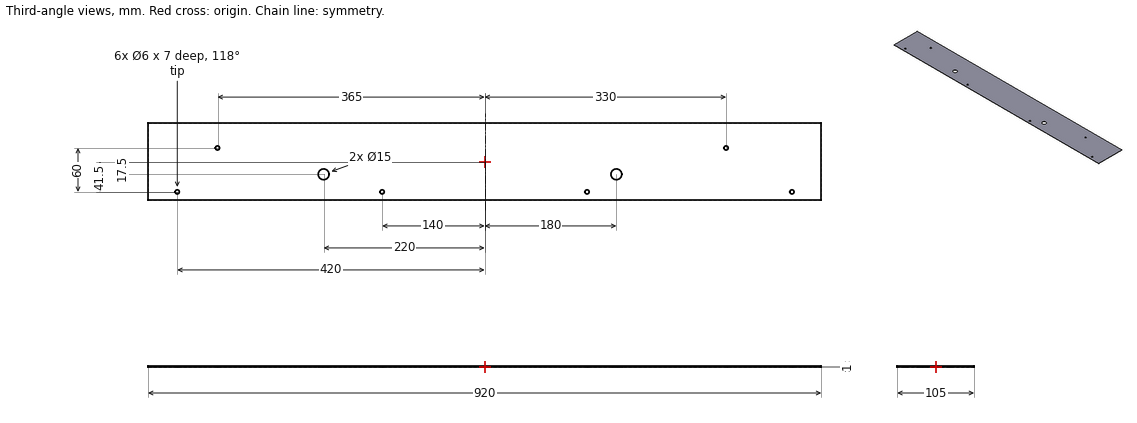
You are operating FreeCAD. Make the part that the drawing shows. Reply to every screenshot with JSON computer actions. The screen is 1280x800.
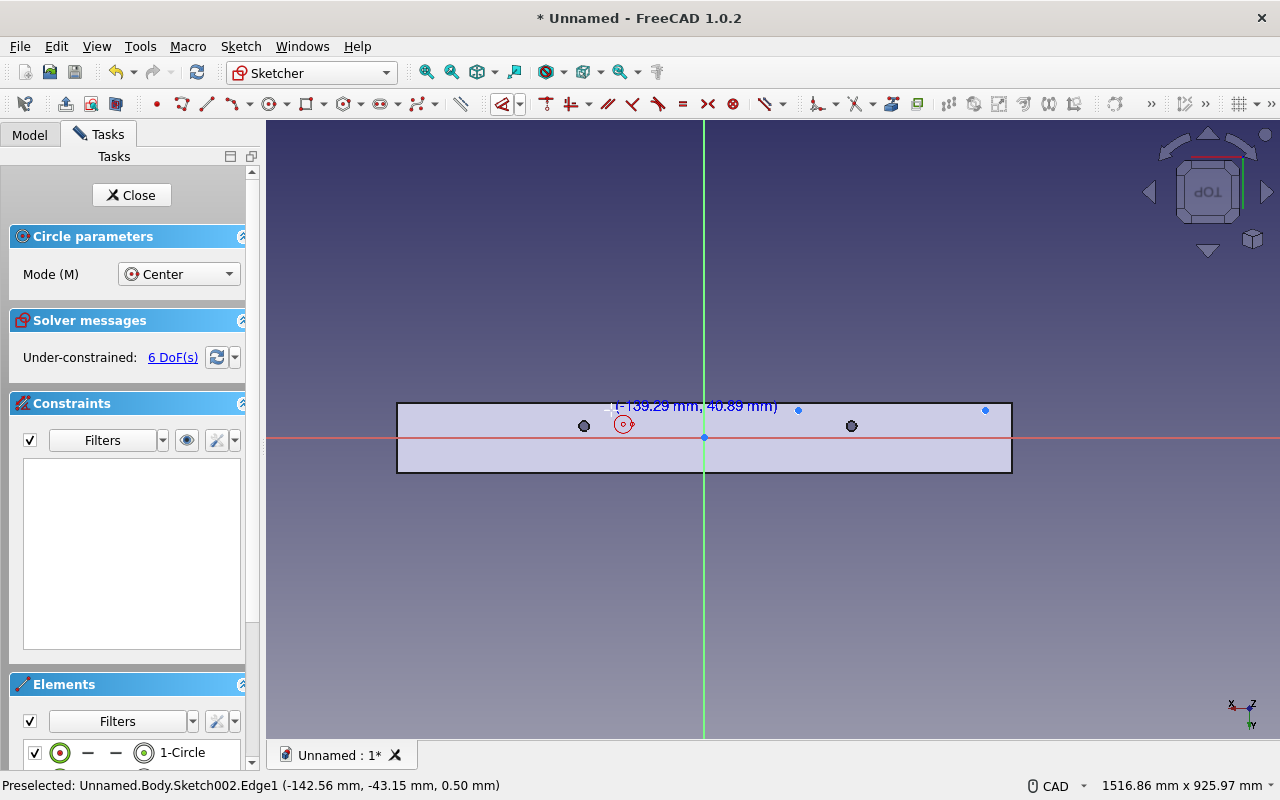
{"action": "left_click", "coordinate": [611, 410]}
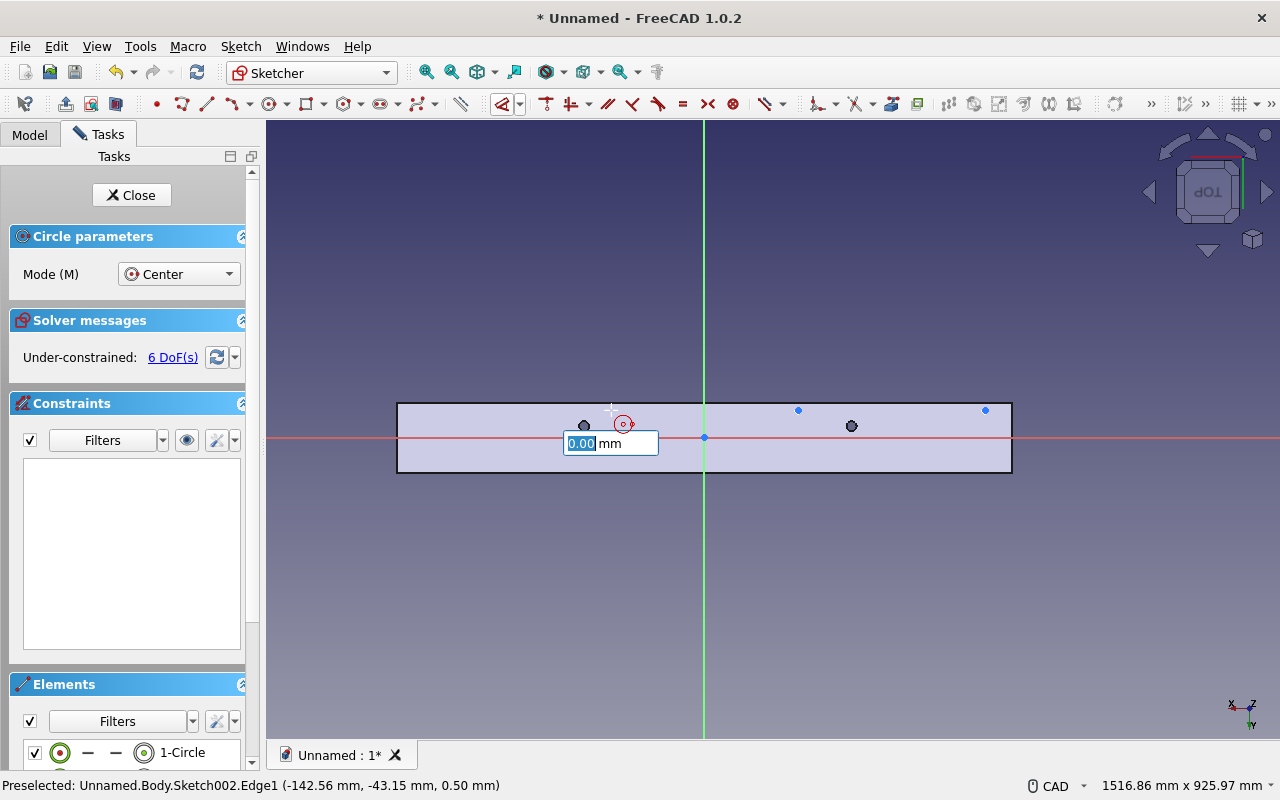
{"action": "scroll", "coordinate": [612, 409], "scroll_direction": "up", "scroll_amount": 11}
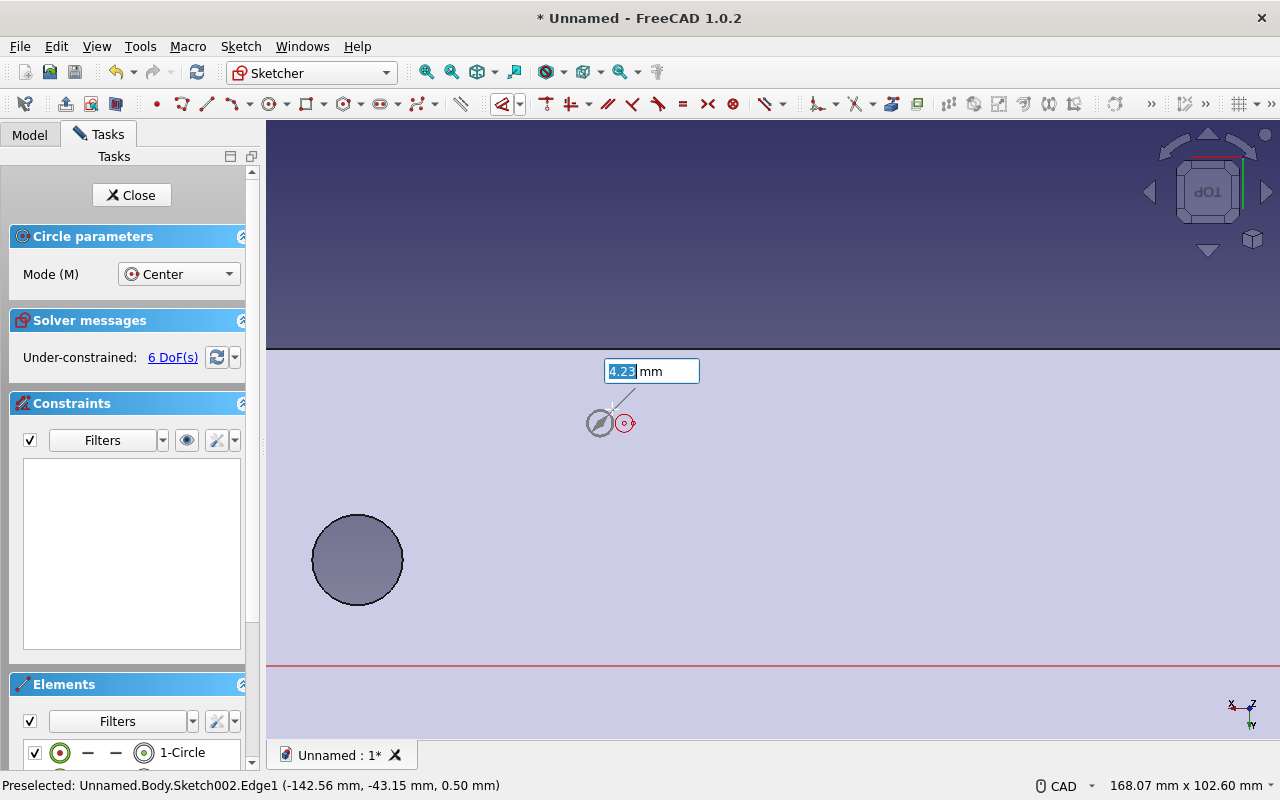
{"action": "left_click", "coordinate": [612, 402]}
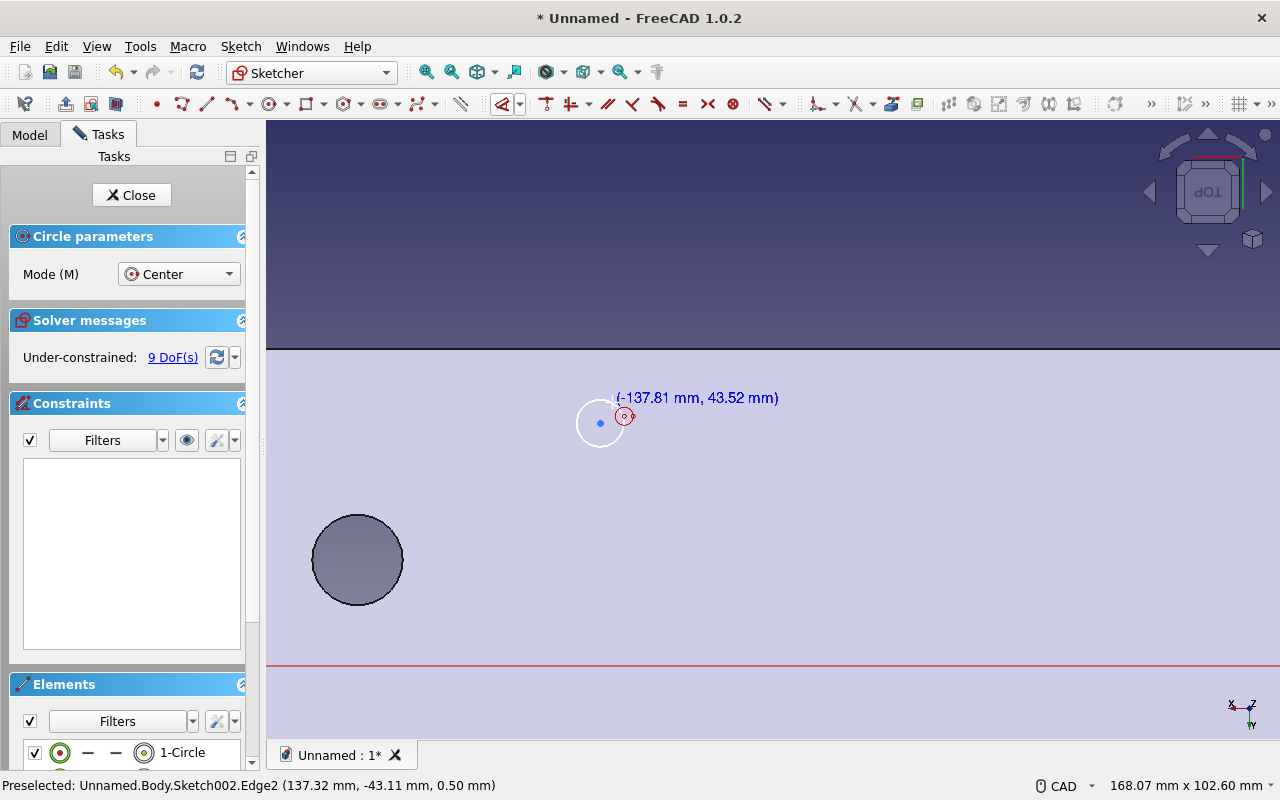
{"action": "scroll", "coordinate": [612, 409], "scroll_direction": "down", "scroll_amount": 11}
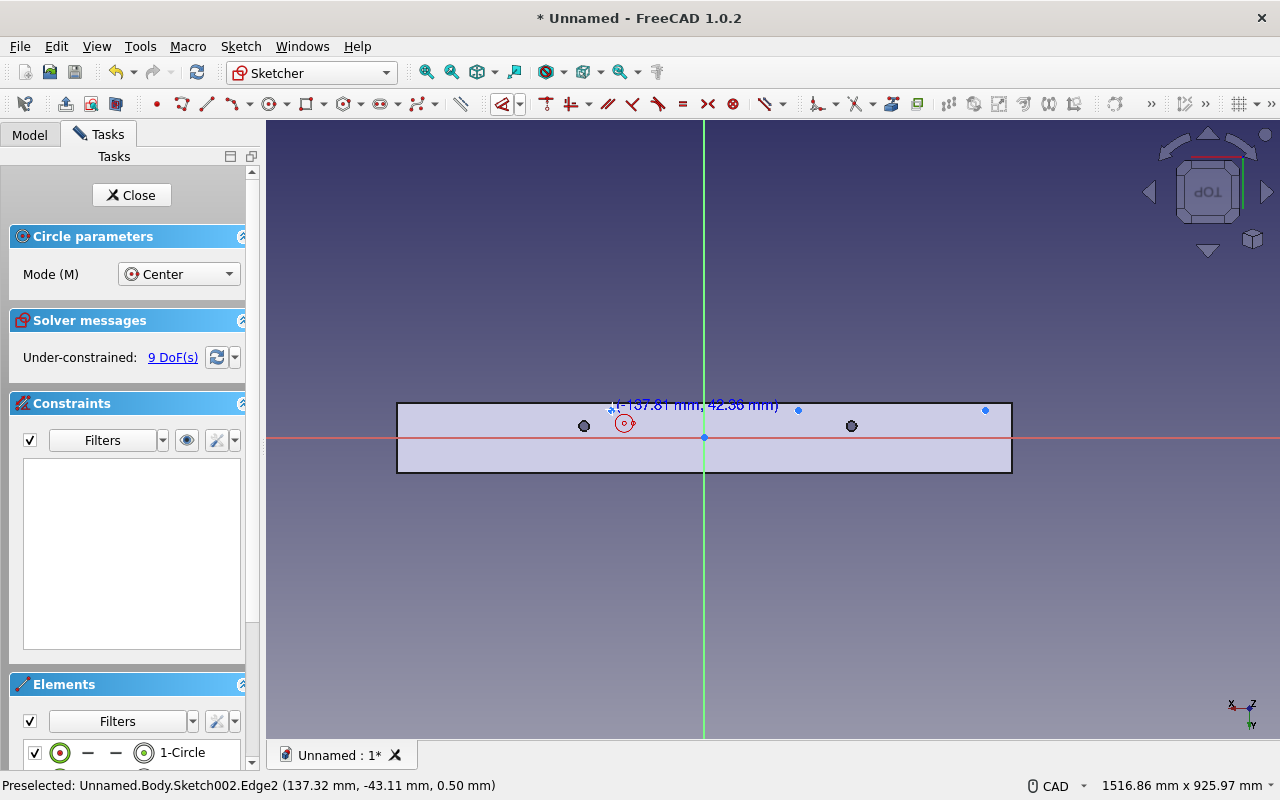
{"action": "scroll", "coordinate": [948, 450], "scroll_direction": "up", "scroll_amount": 13}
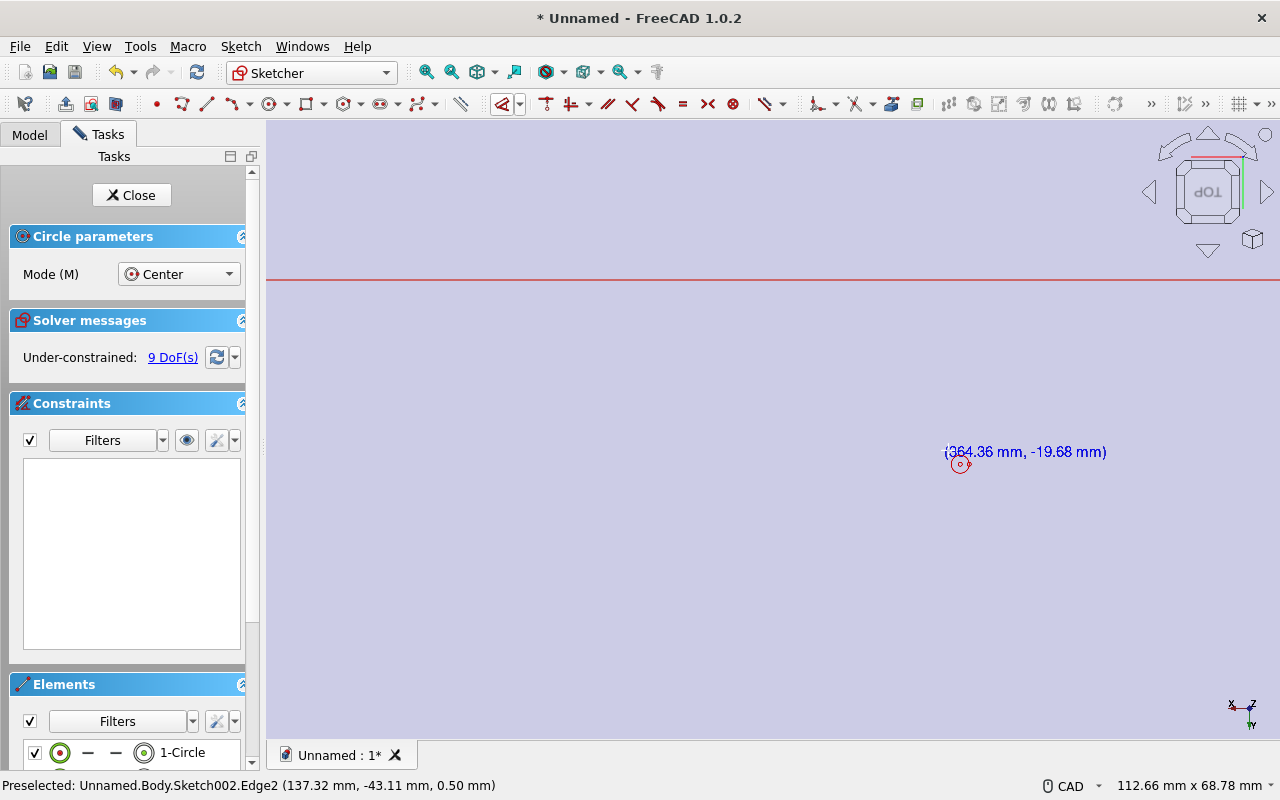
{"action": "scroll", "coordinate": [949, 450], "scroll_direction": "down", "scroll_amount": 13}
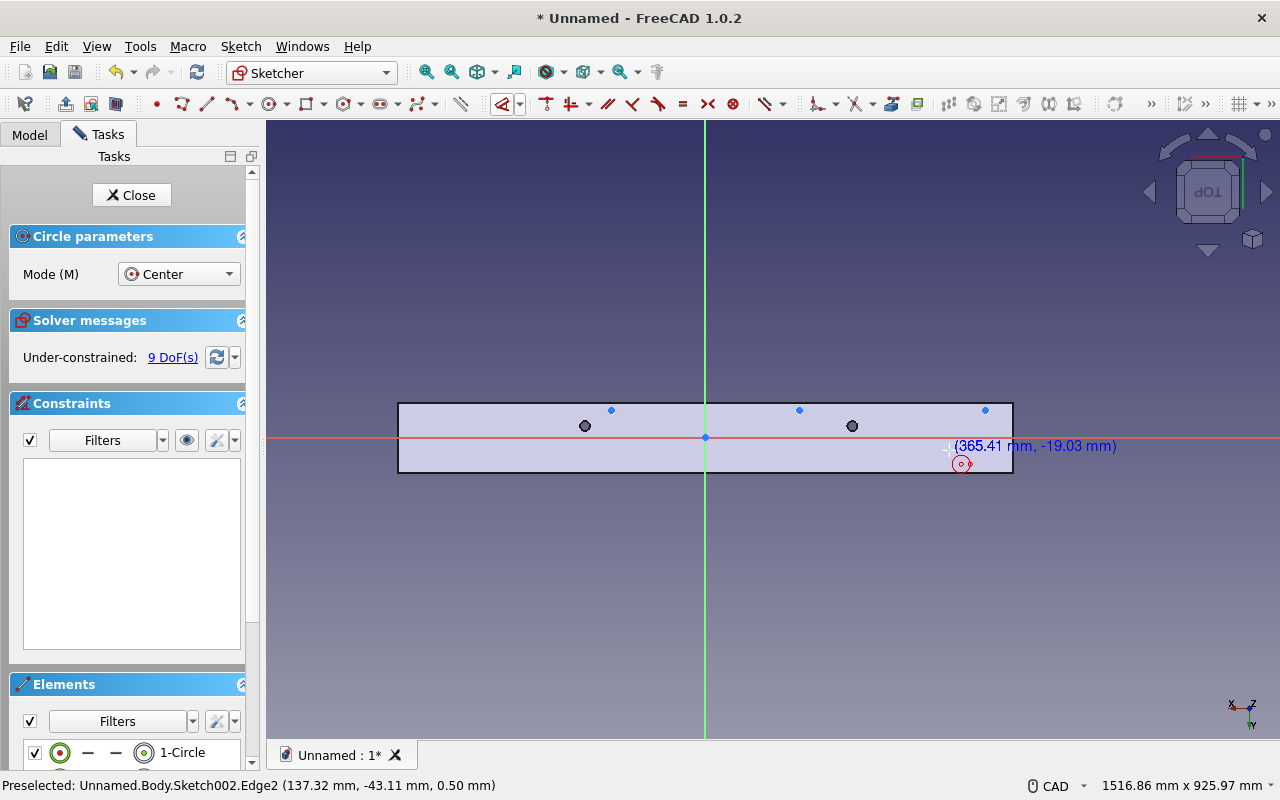
{"action": "scroll", "coordinate": [949, 450], "scroll_direction": "up", "scroll_amount": 2}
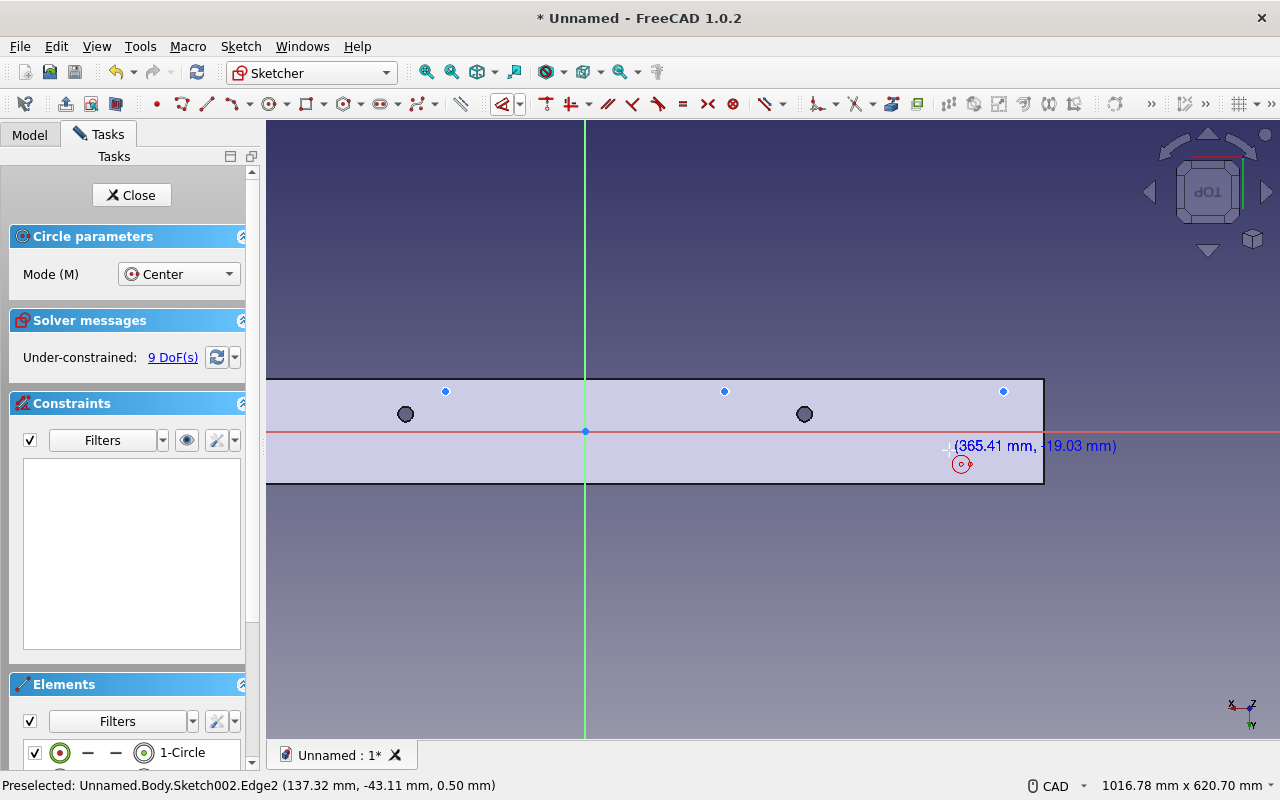
{"action": "left_click", "coordinate": [949, 450]}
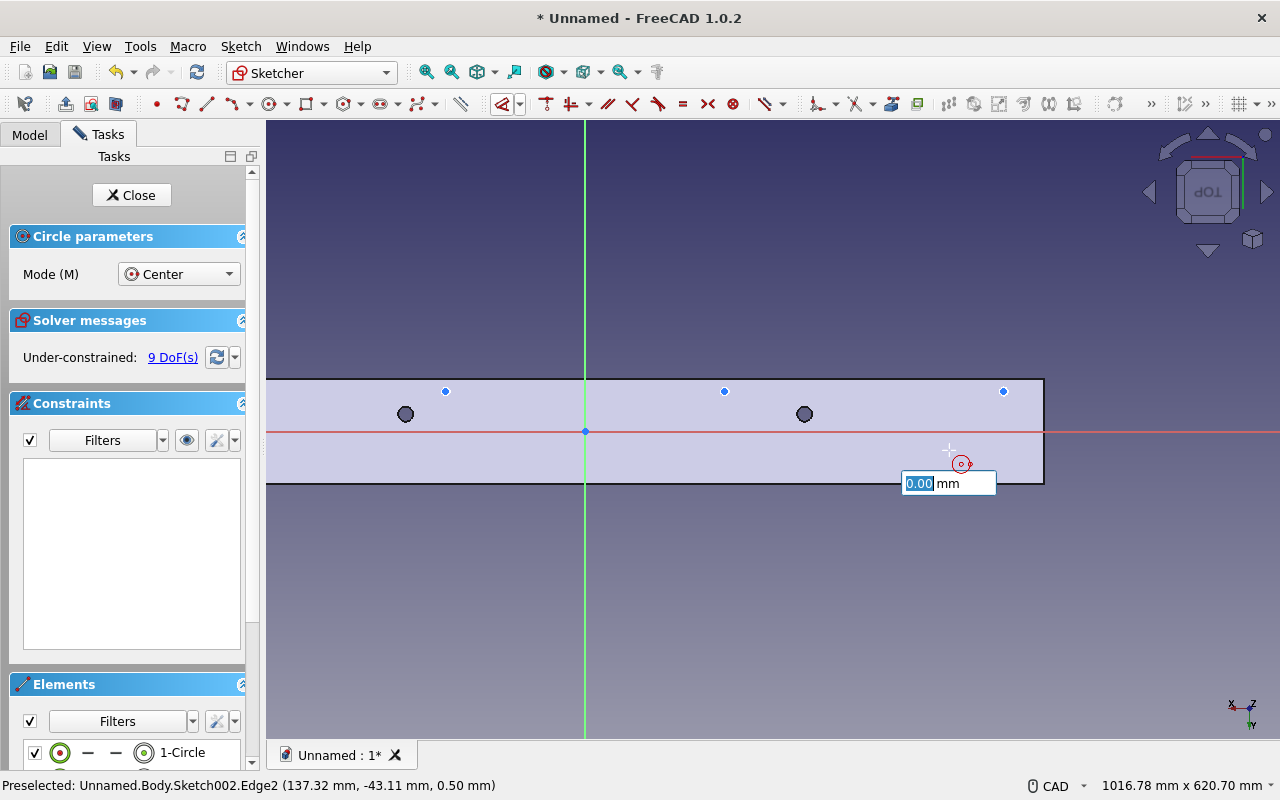
{"action": "scroll", "coordinate": [951, 448], "scroll_direction": "up", "scroll_amount": 9}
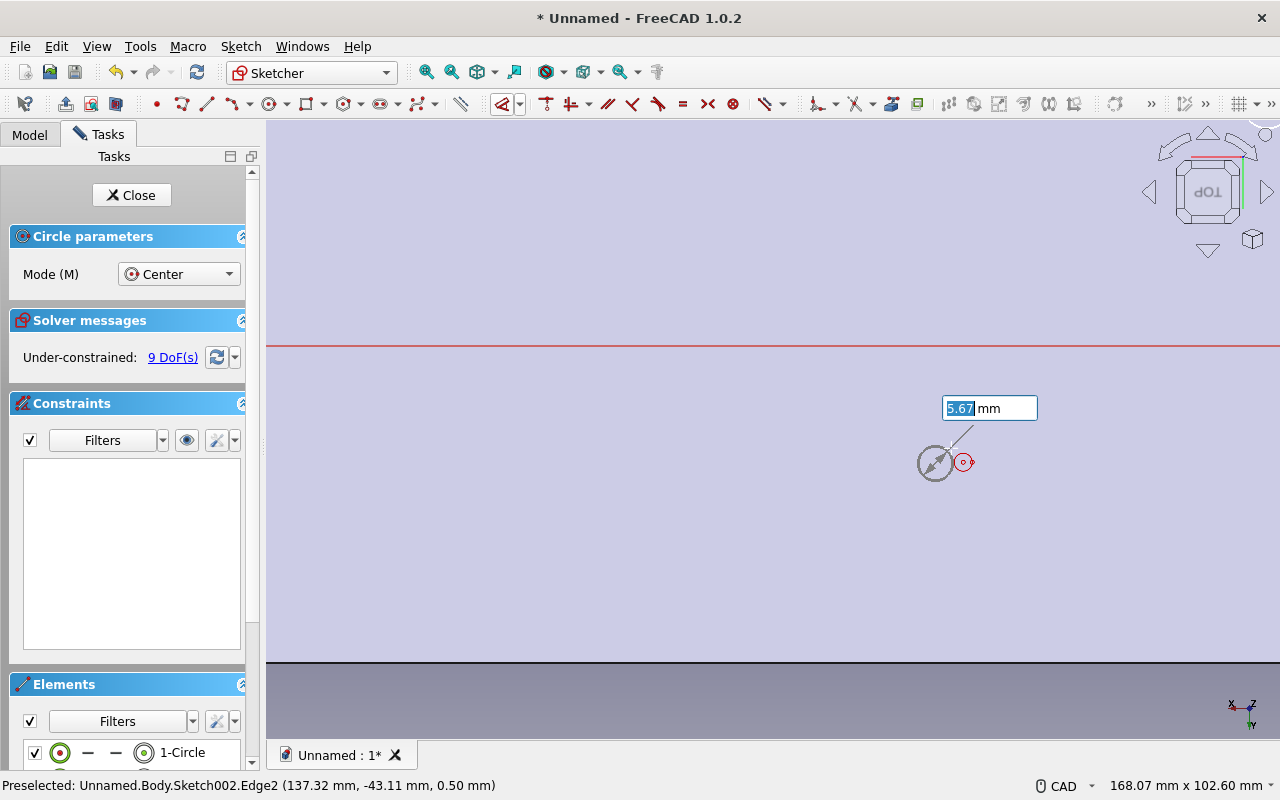
{"action": "left_click", "coordinate": [949, 445]}